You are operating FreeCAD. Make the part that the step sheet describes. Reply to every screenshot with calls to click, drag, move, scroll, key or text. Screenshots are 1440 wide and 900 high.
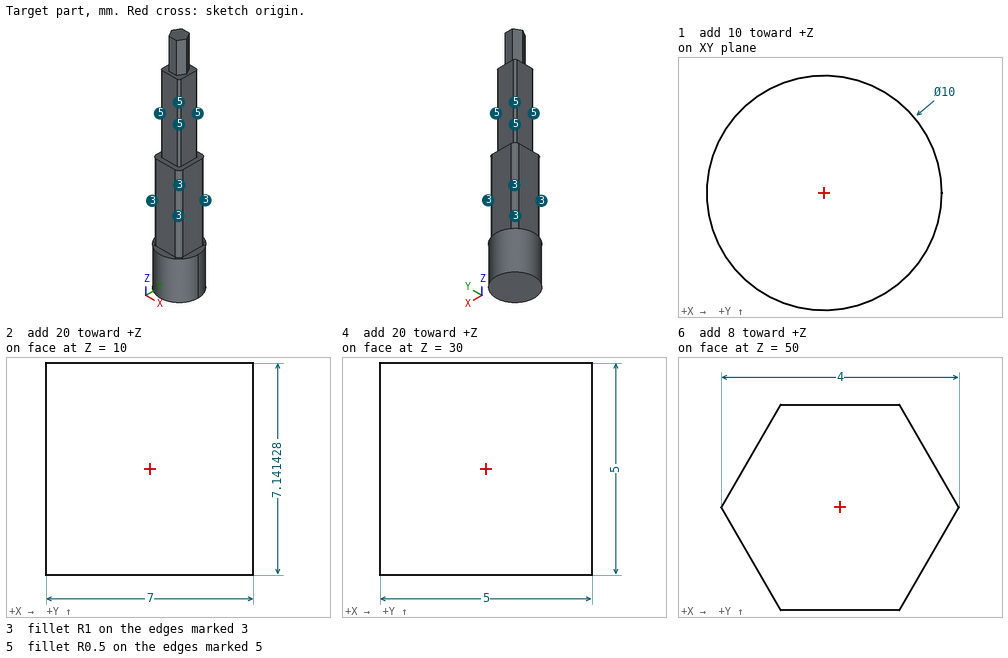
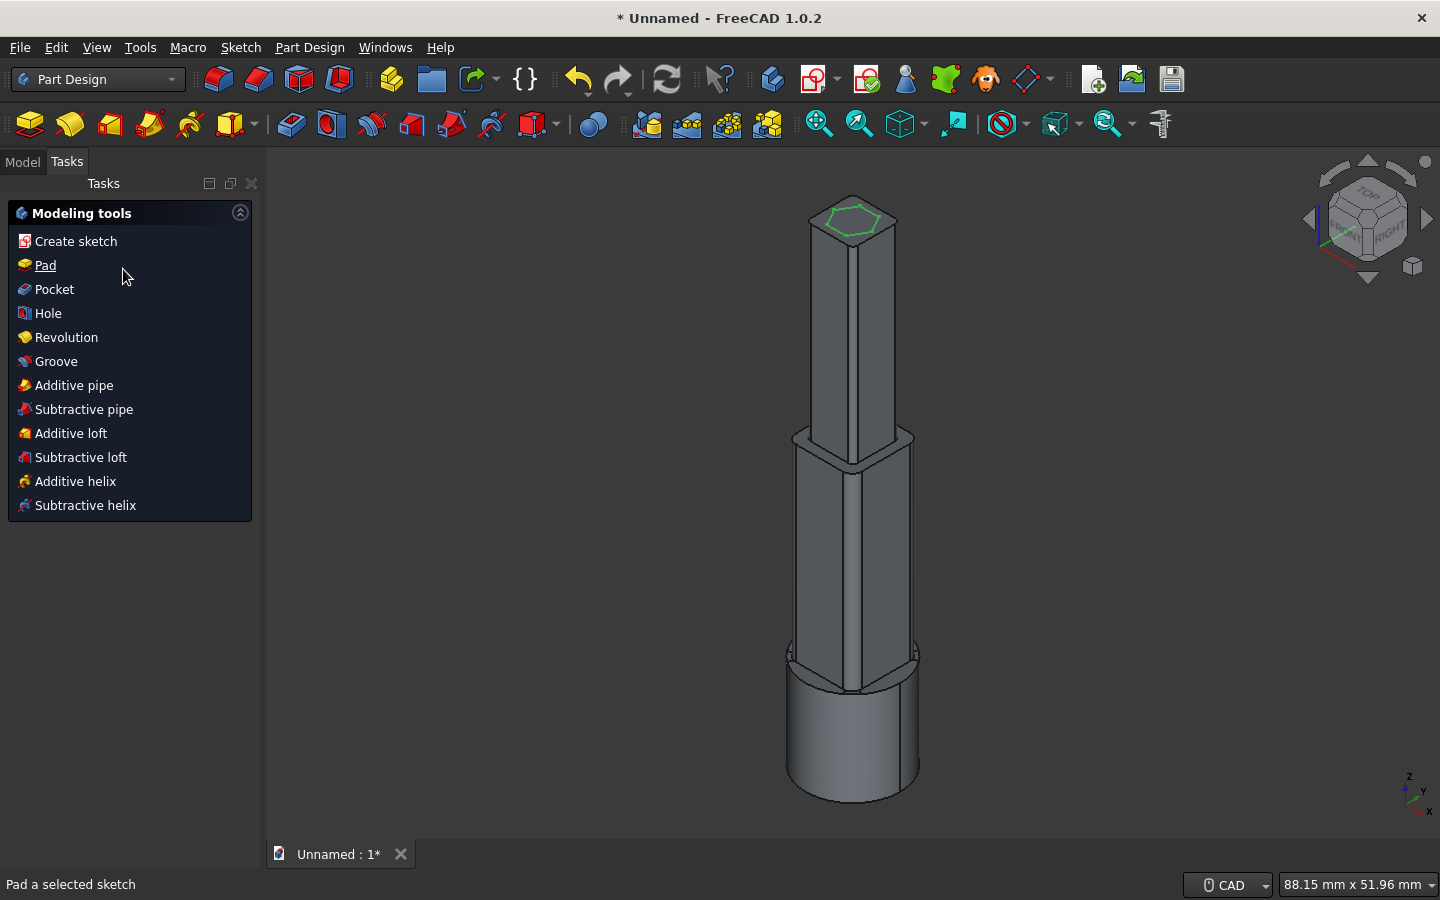
click(30, 124)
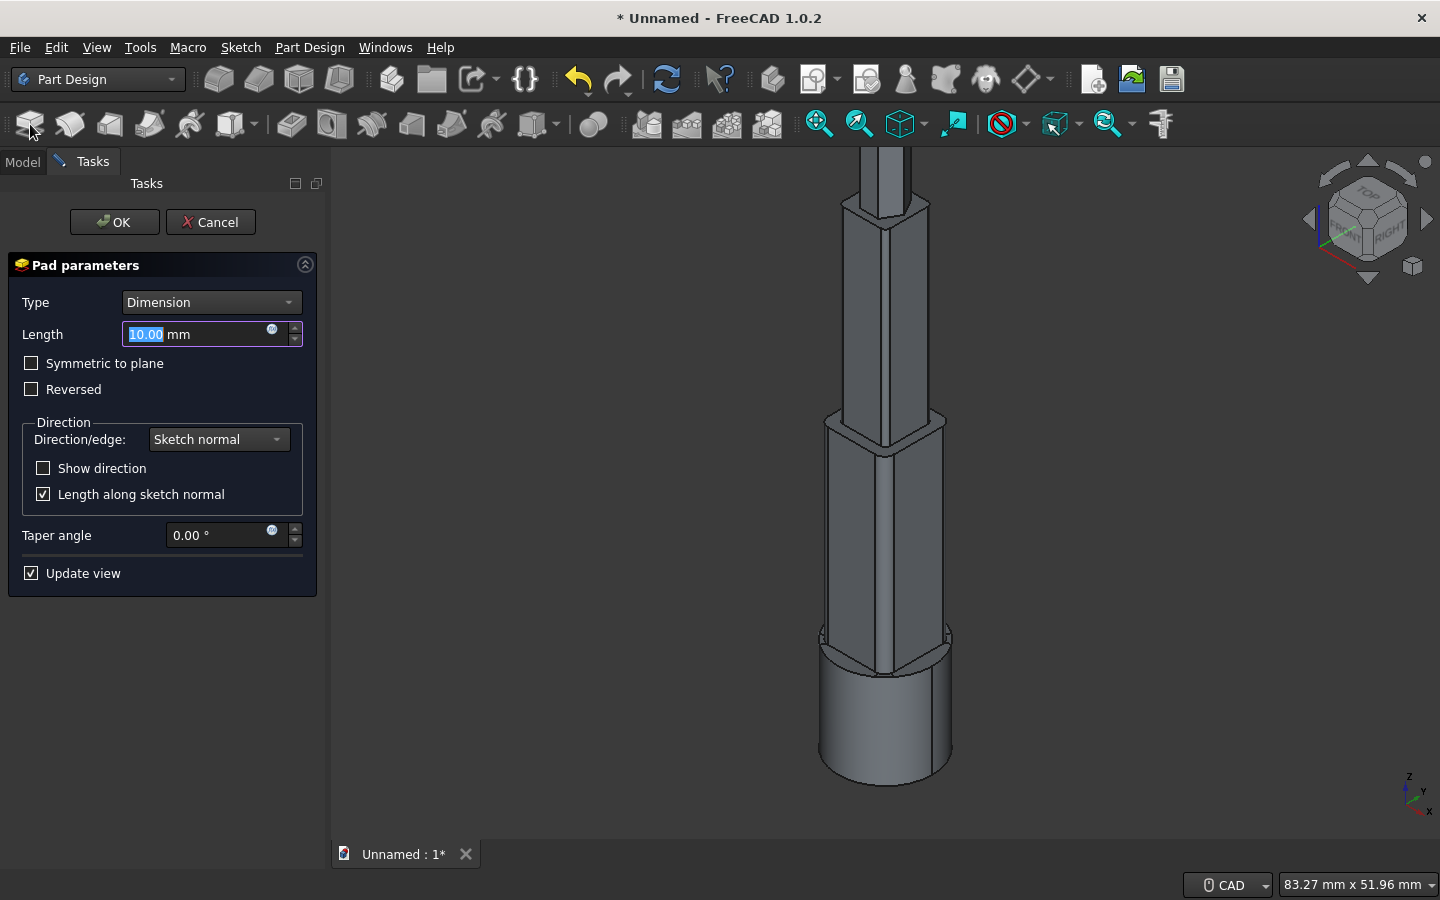
text(8)
key(Tab)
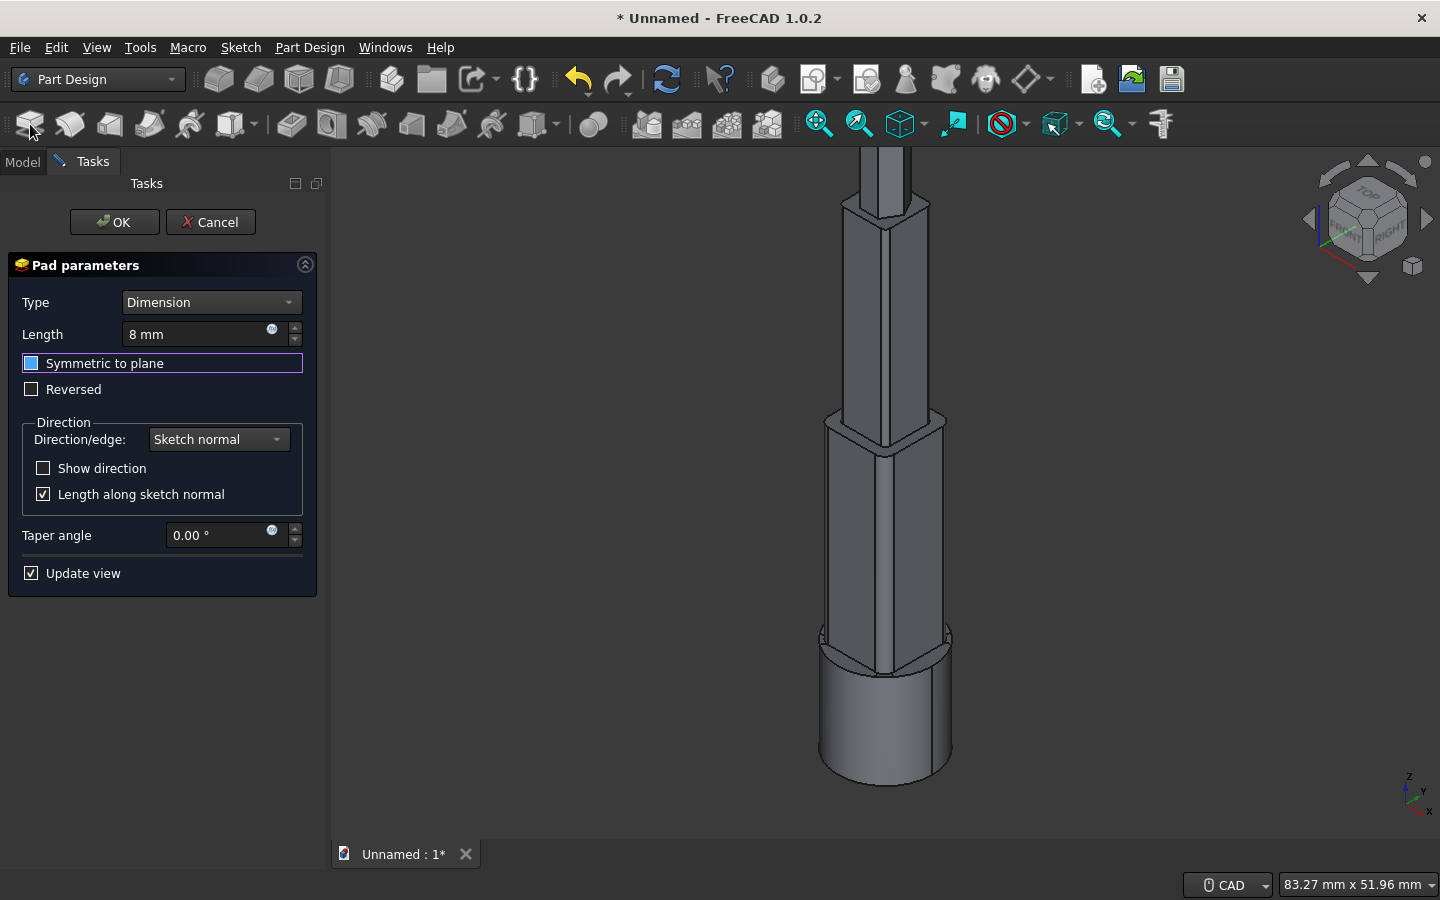
click(115, 222)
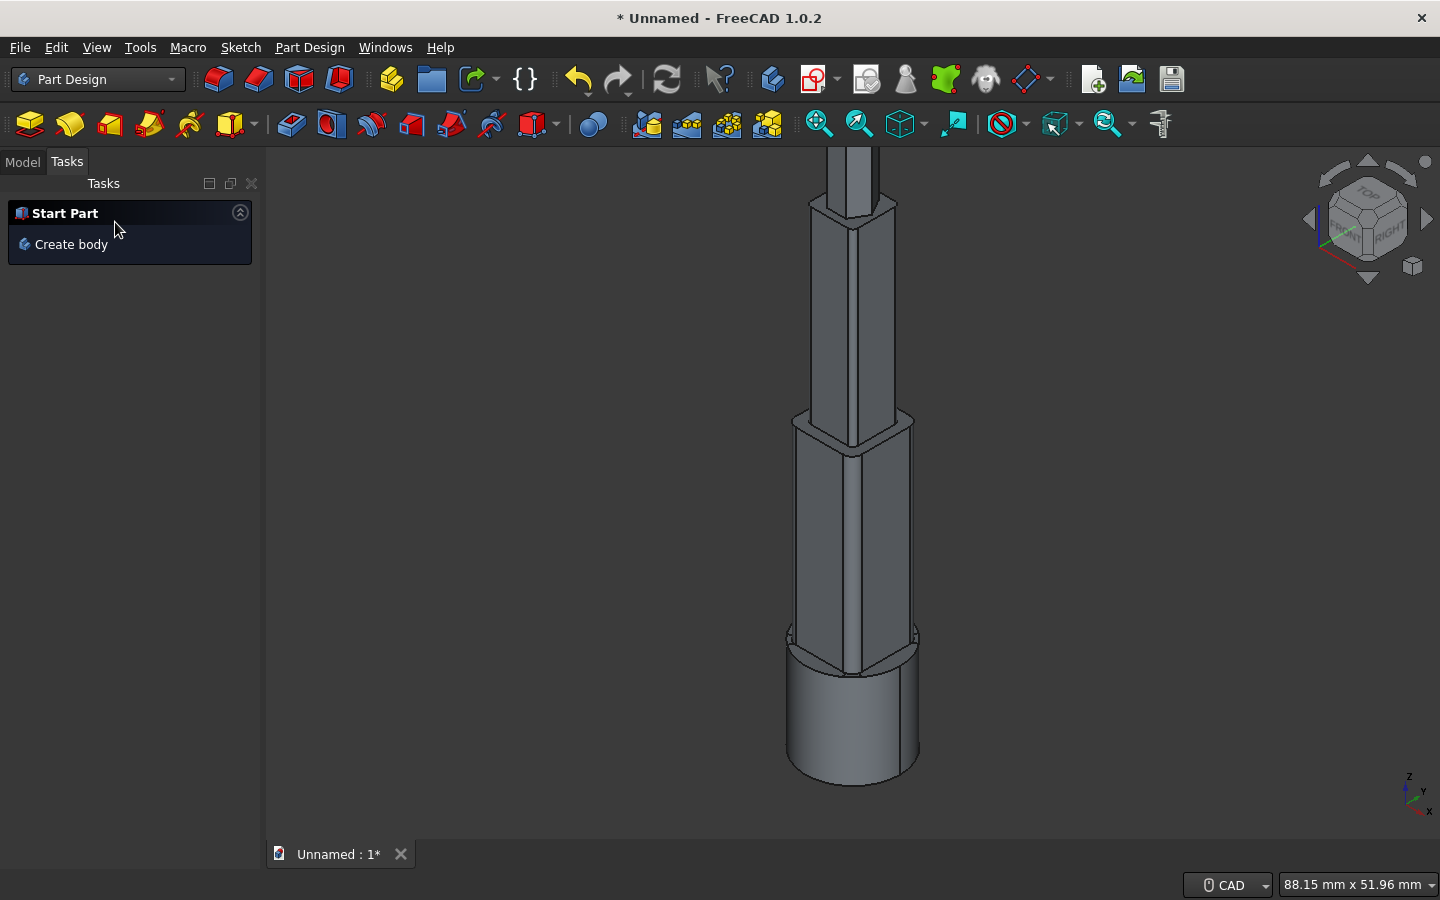
click(820, 124)